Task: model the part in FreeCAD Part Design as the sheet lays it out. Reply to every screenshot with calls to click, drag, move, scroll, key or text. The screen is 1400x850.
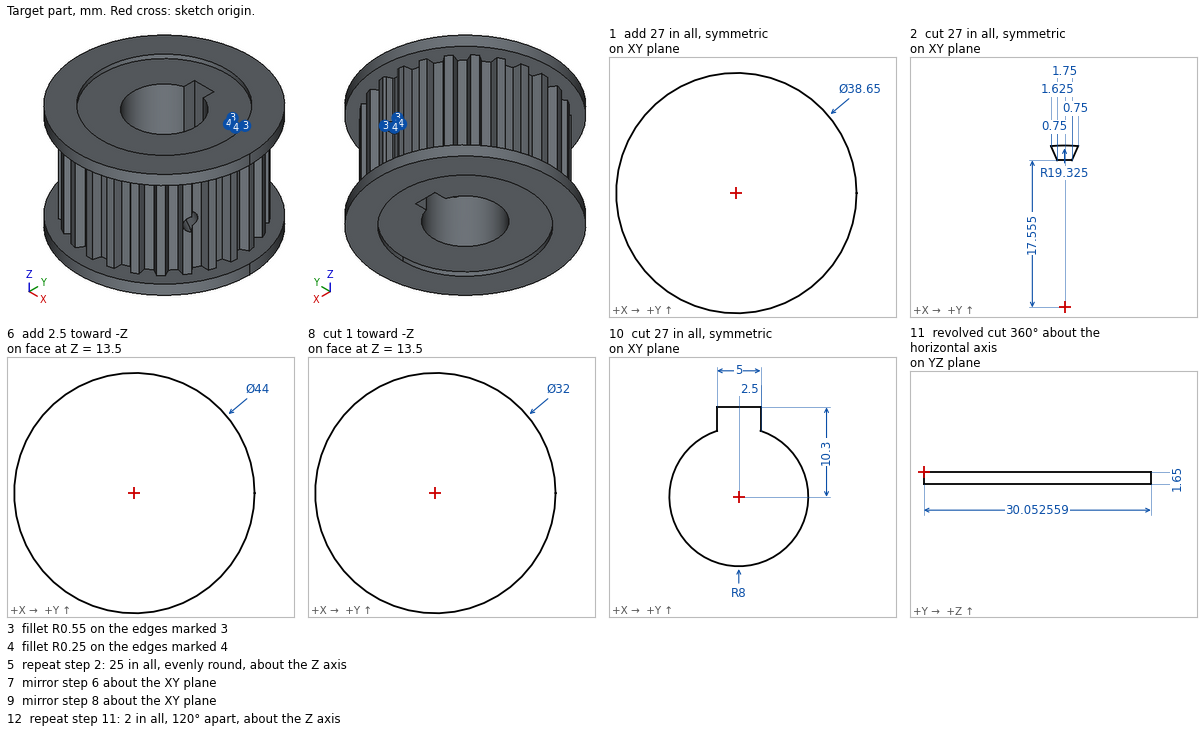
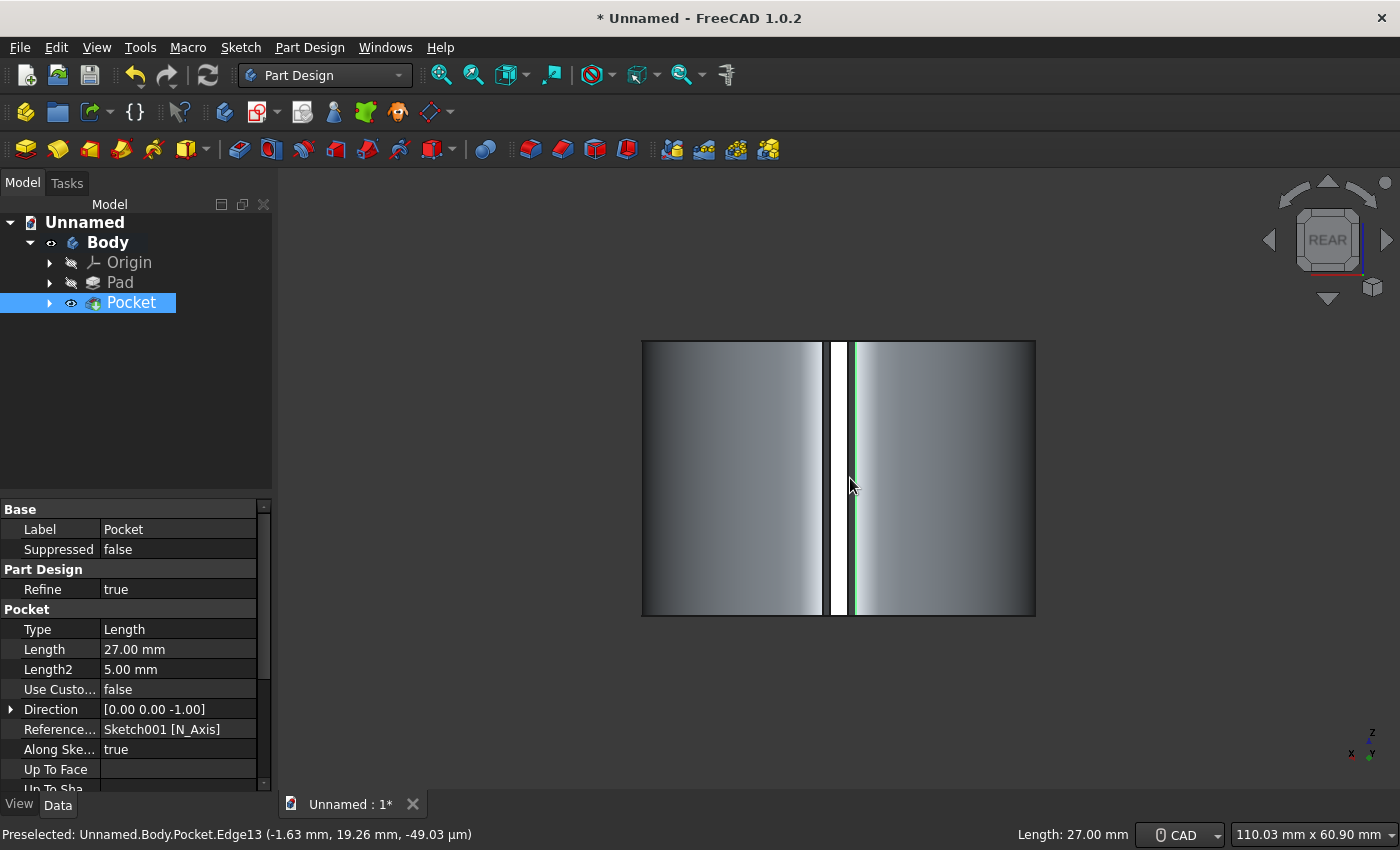
click(823, 478, ctrl)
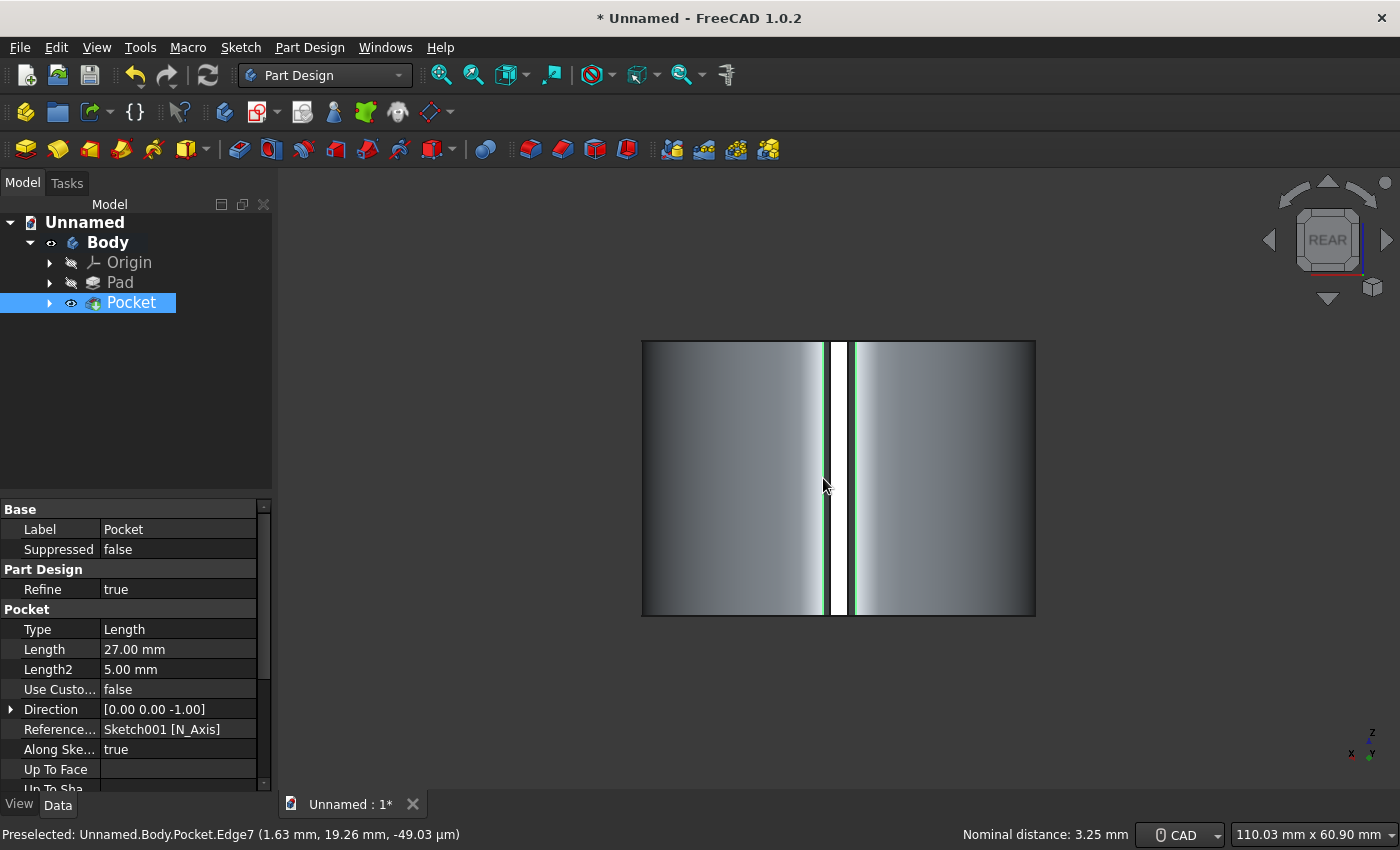
click(532, 150)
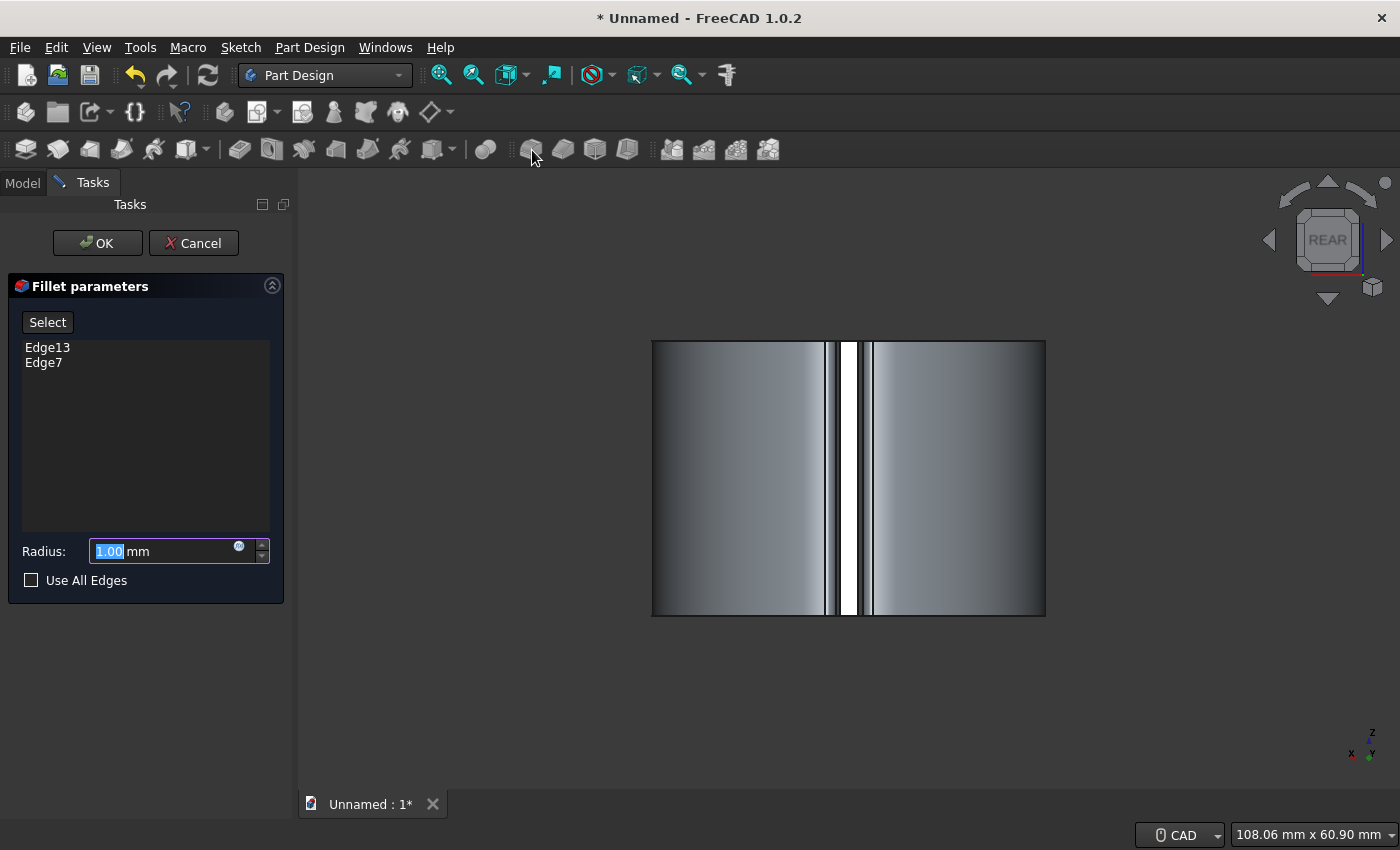
text(0.55)
key(Tab)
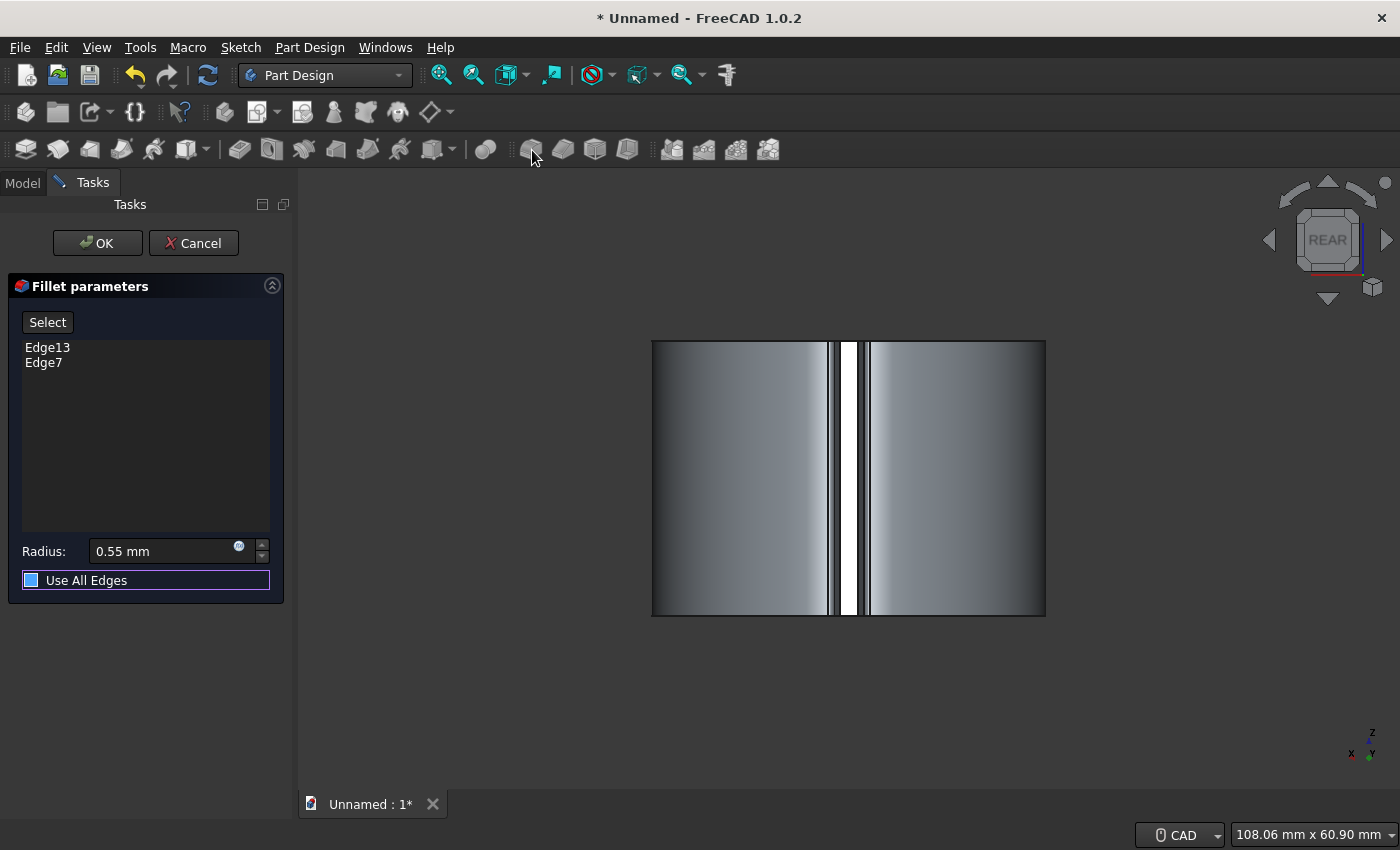
click(98, 243)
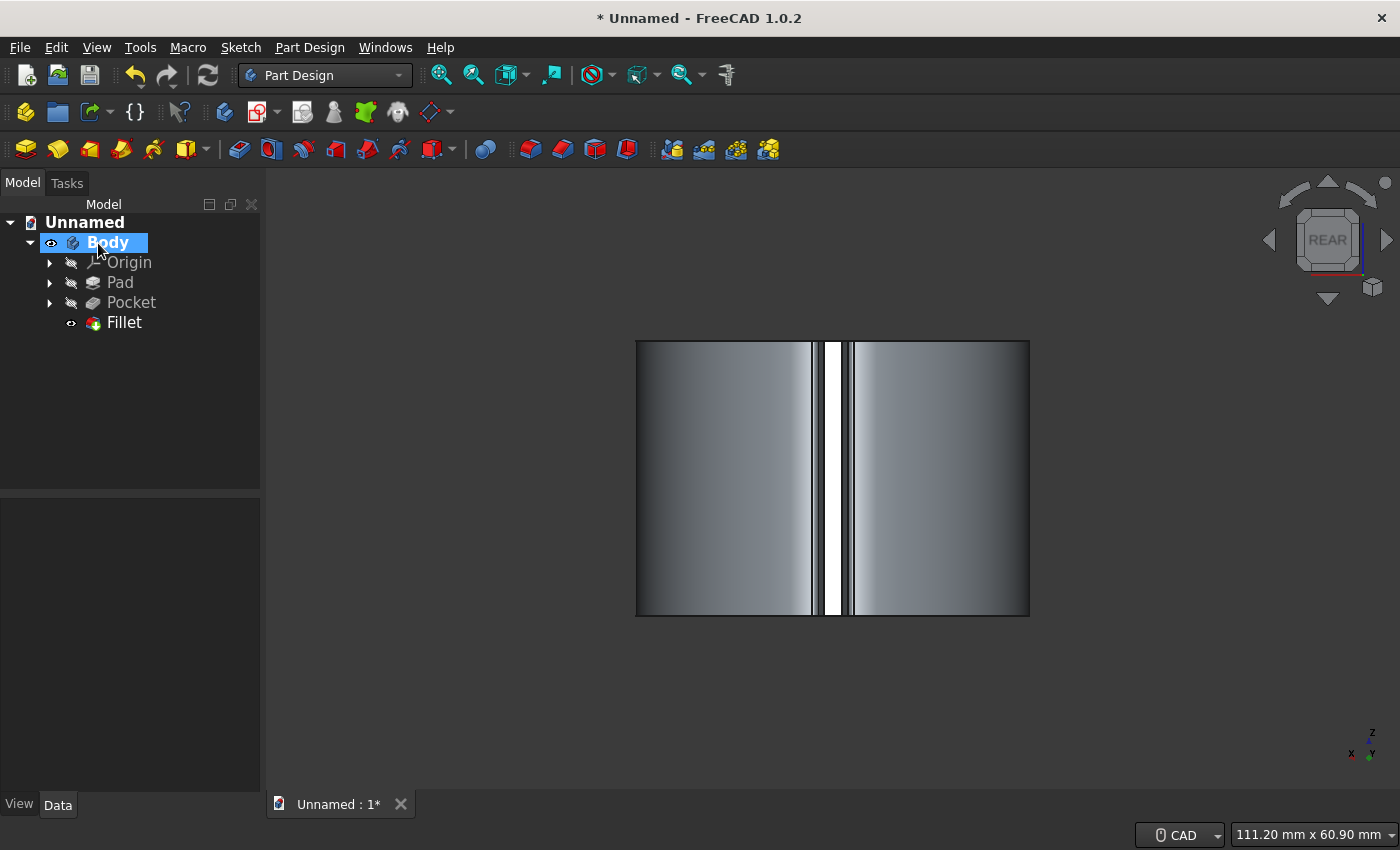
click(442, 76)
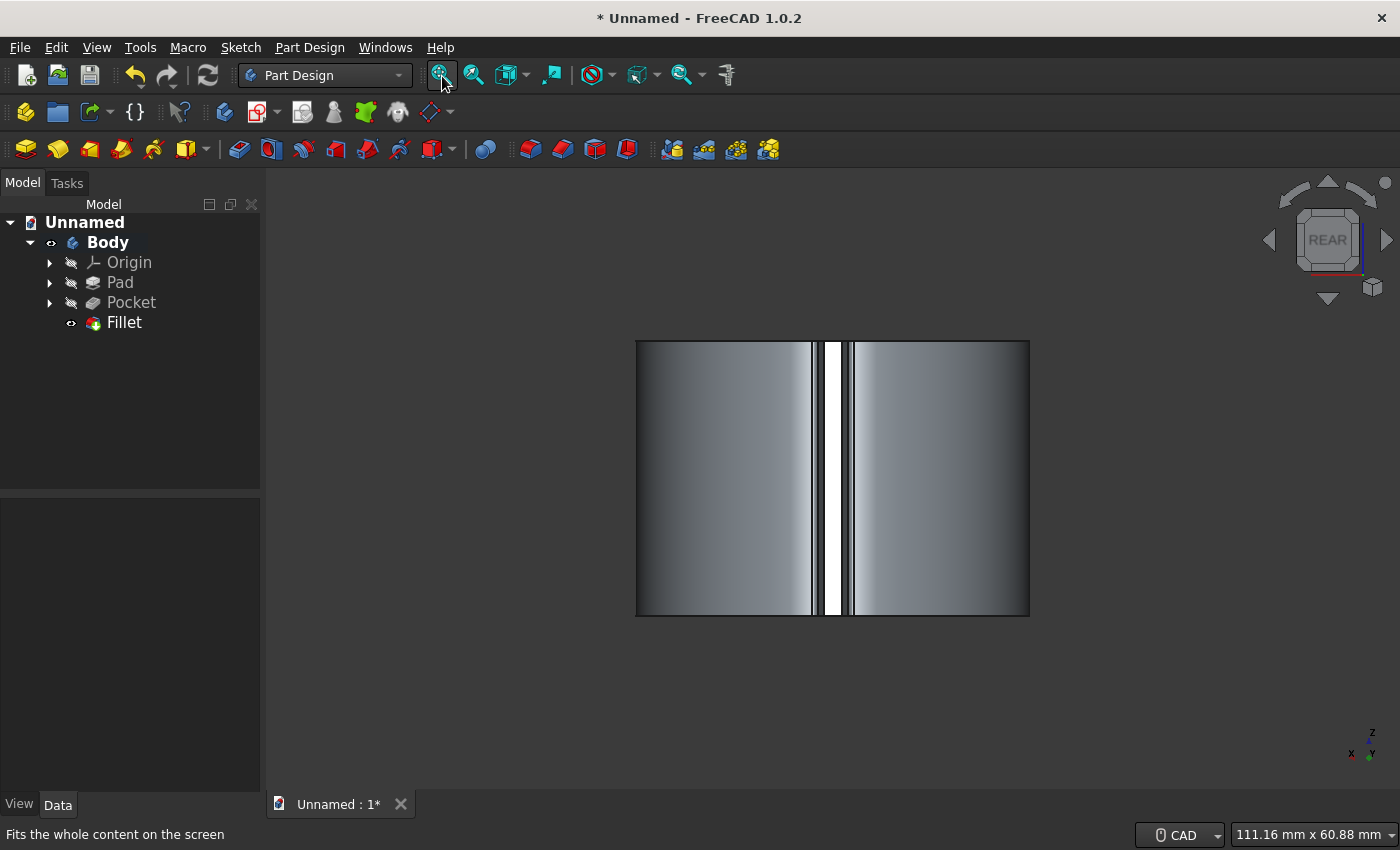
key(0)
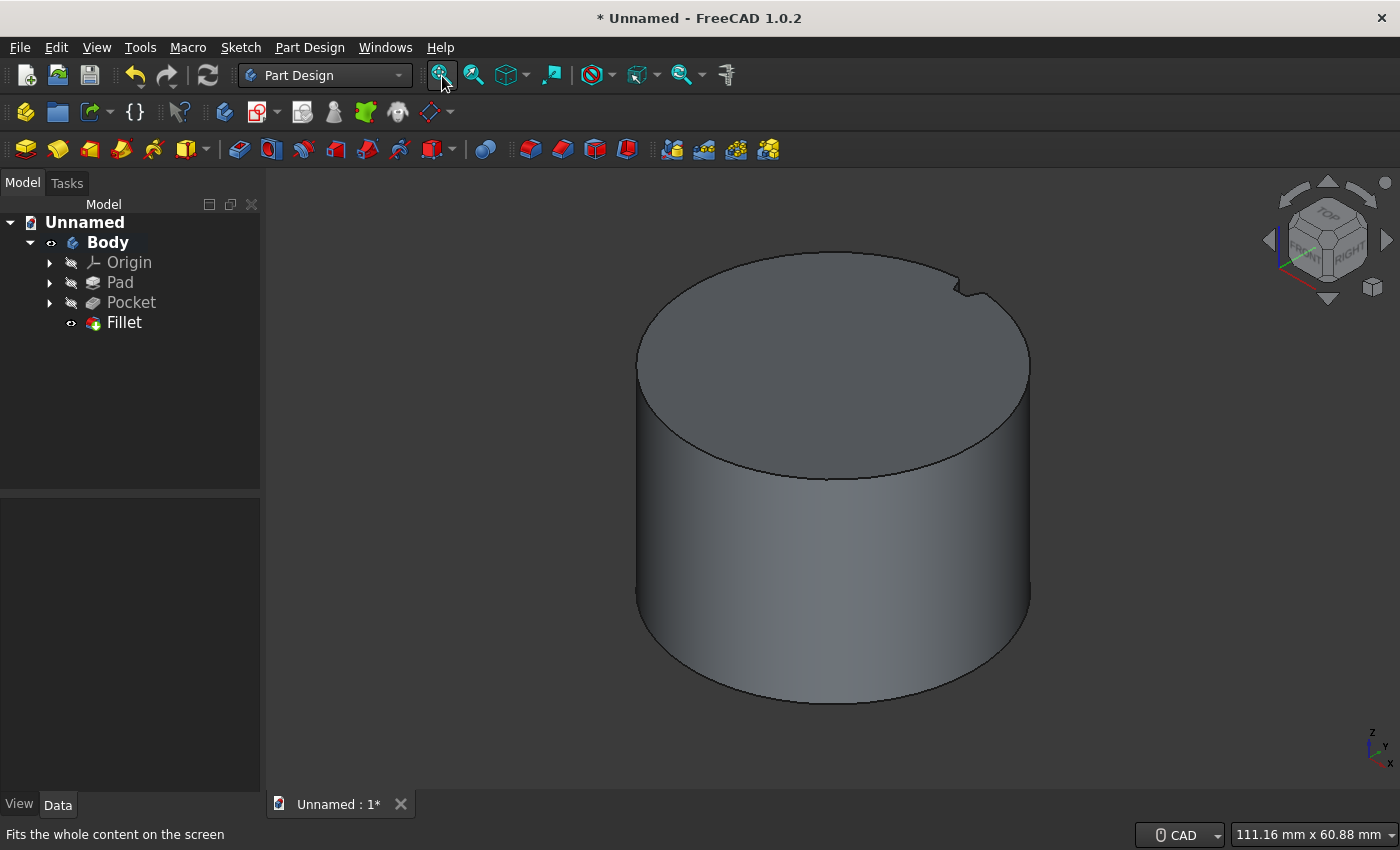
key(2)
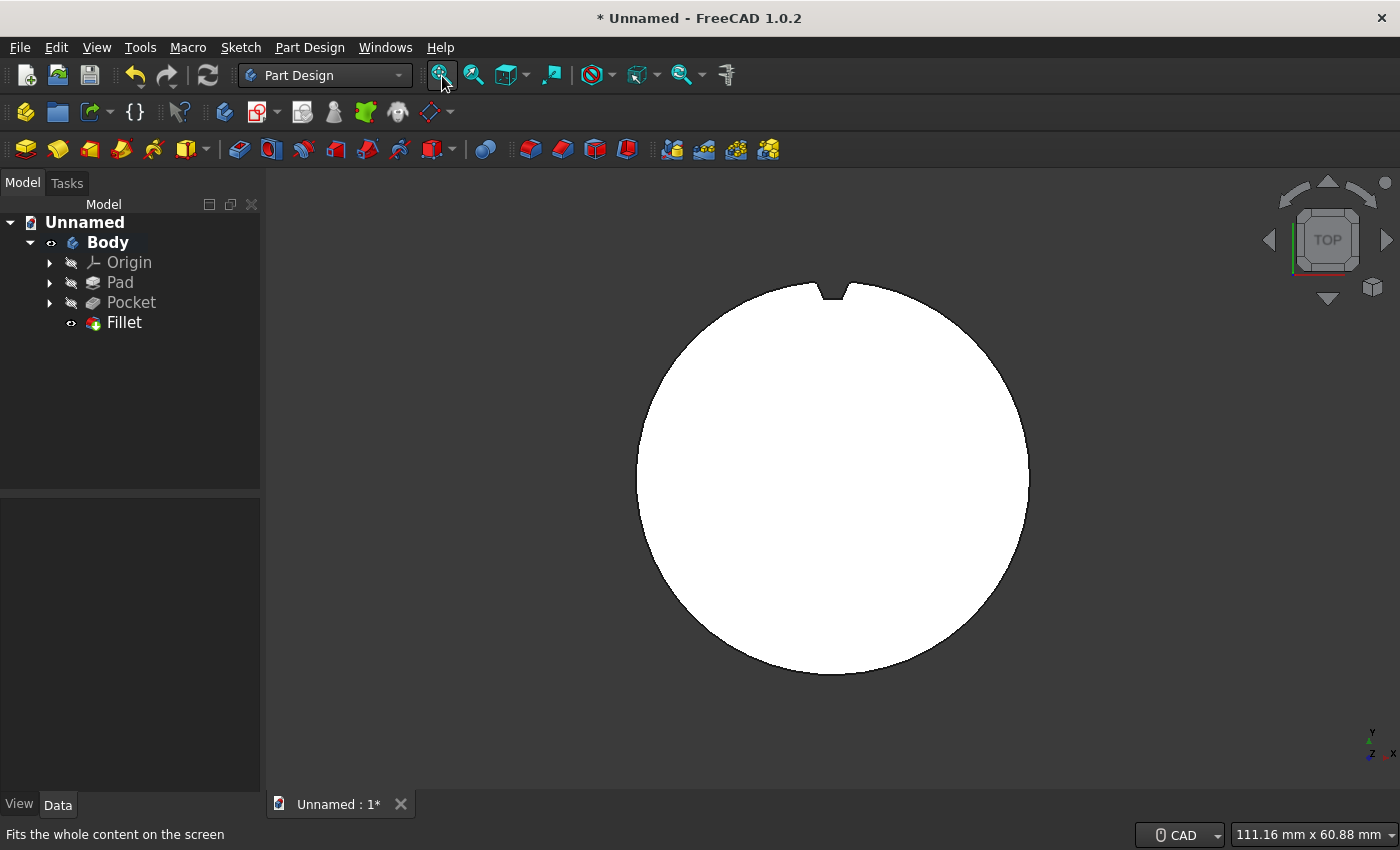
key(1)